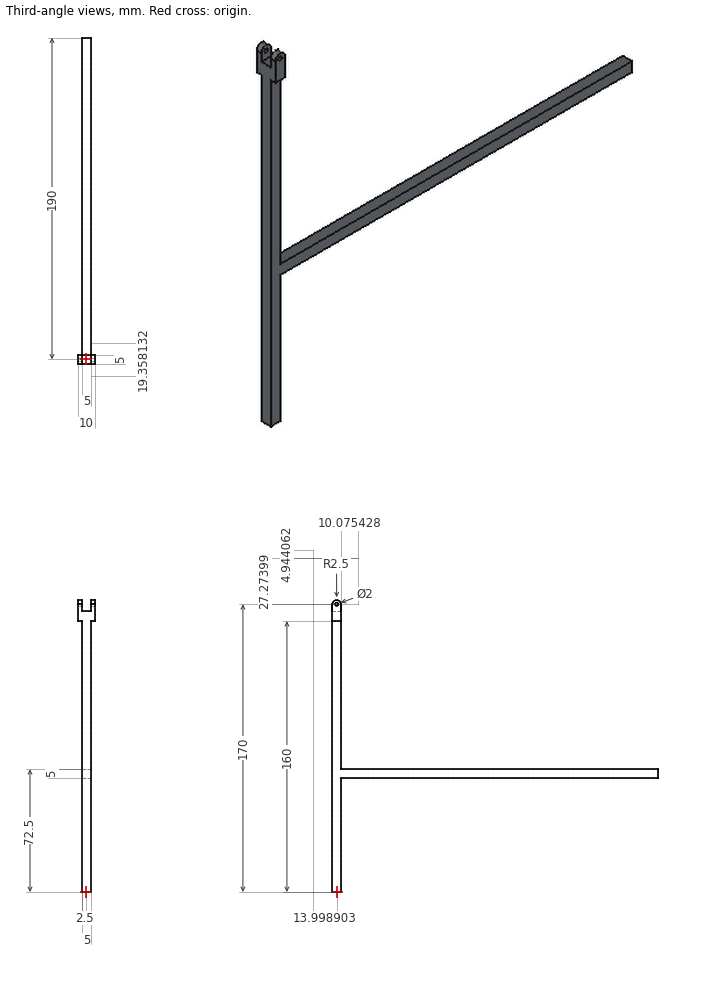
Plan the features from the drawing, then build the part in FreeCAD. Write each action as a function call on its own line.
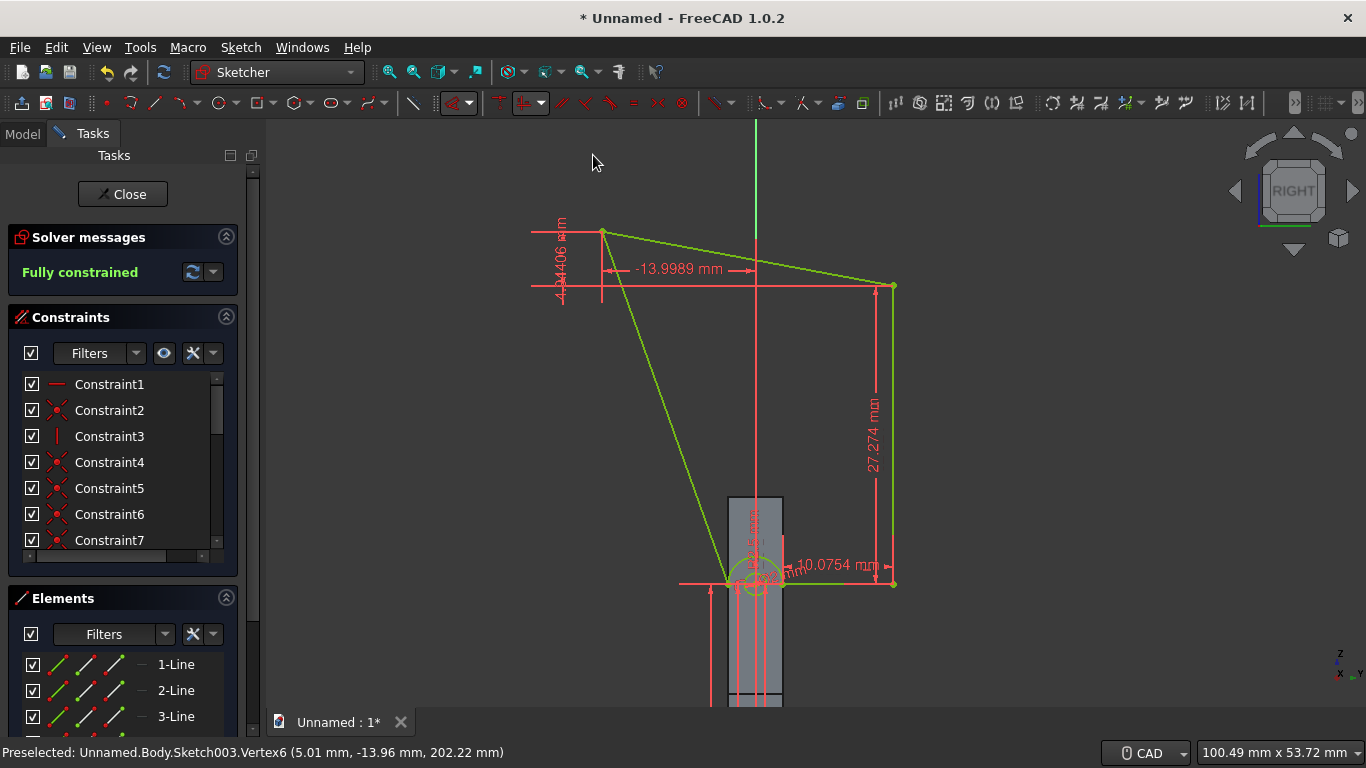
click(123, 194)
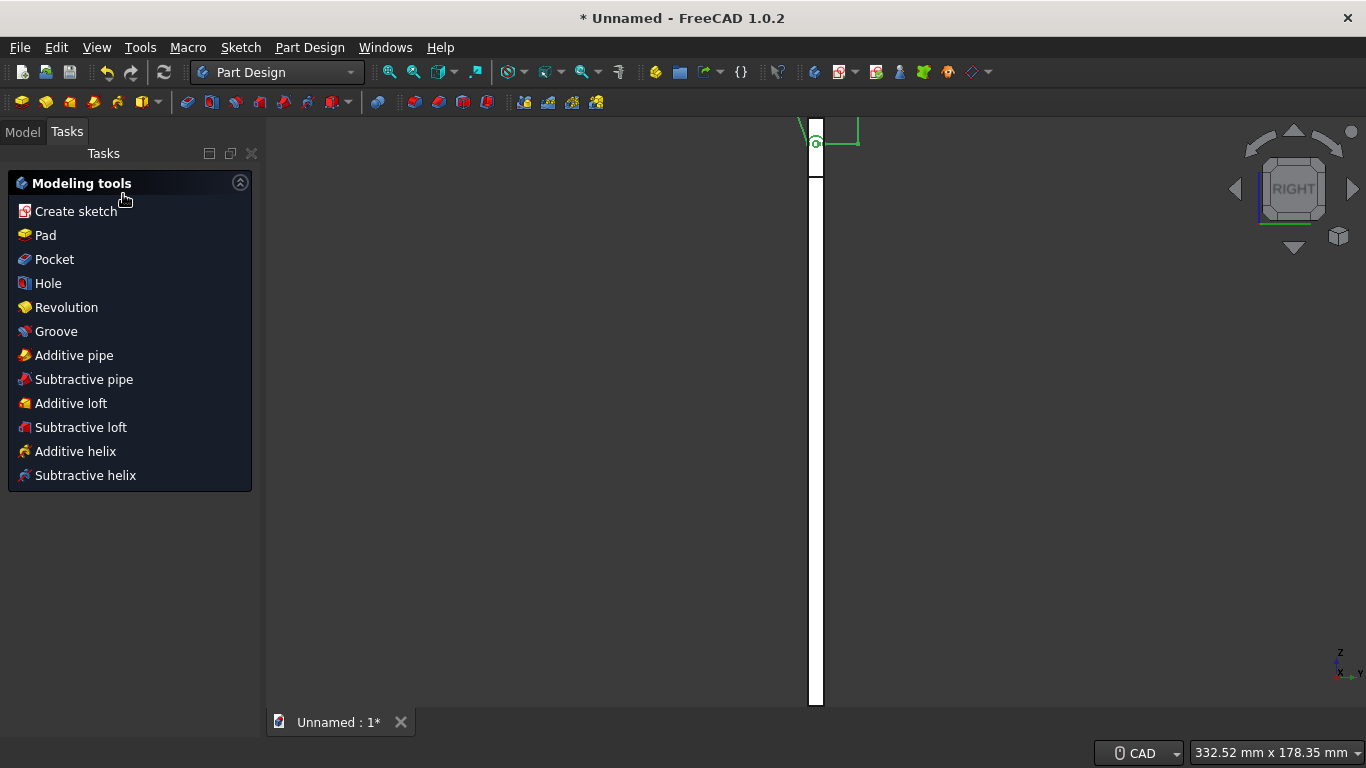
click(188, 102)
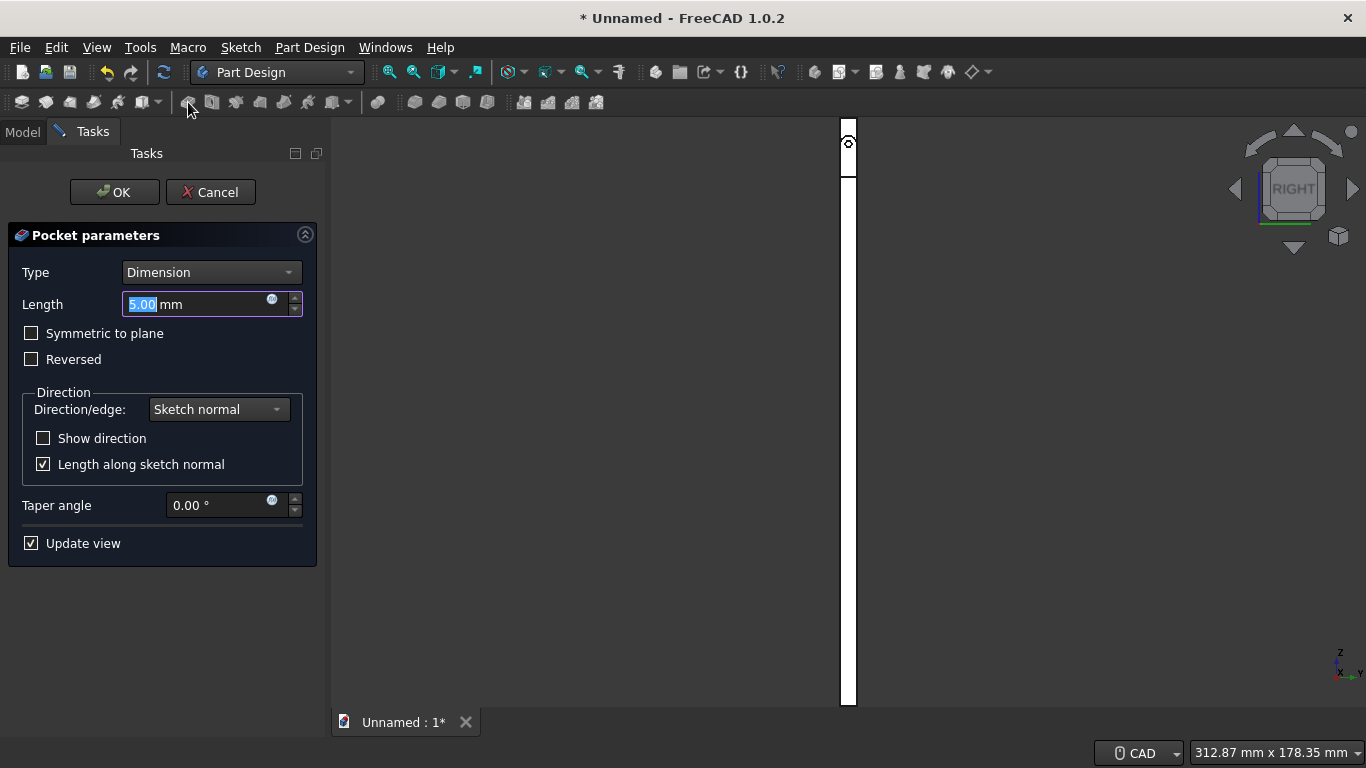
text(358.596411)
key(Tab)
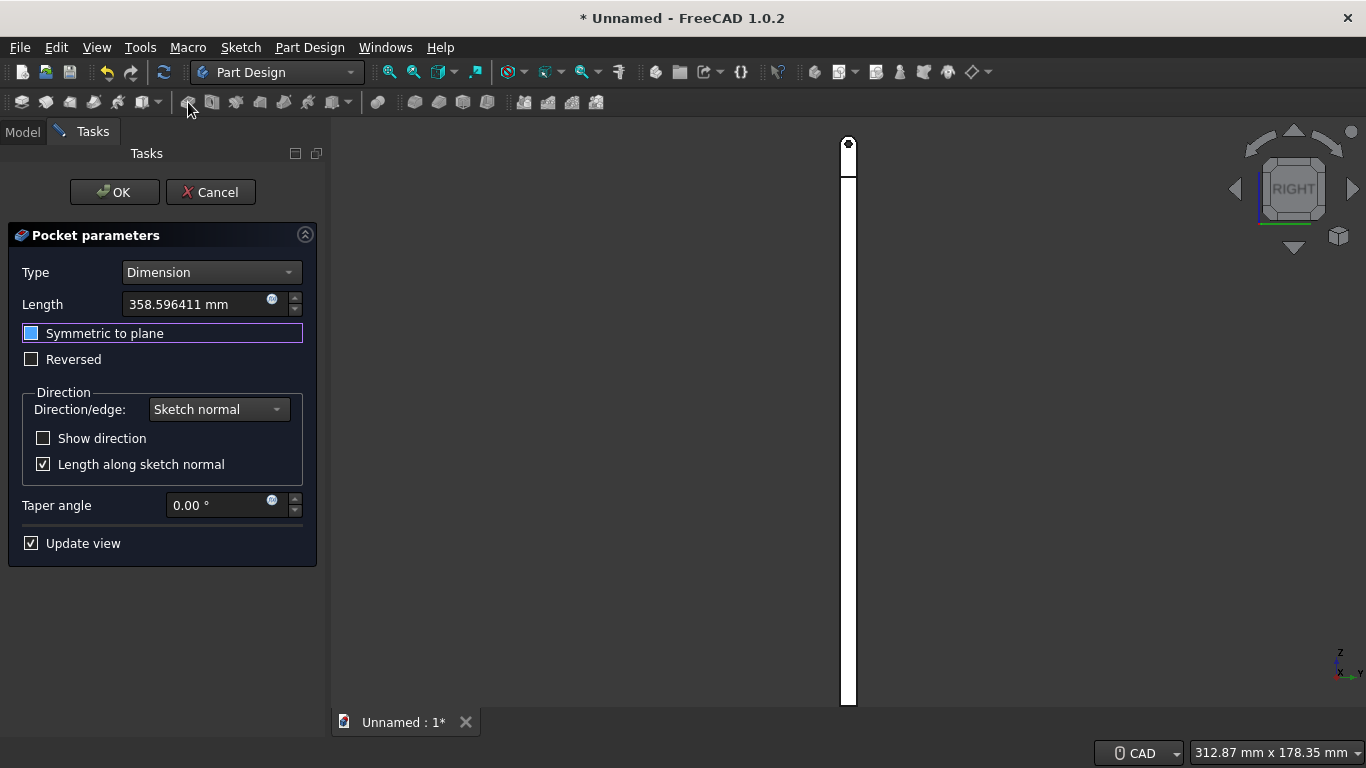
click(30, 333)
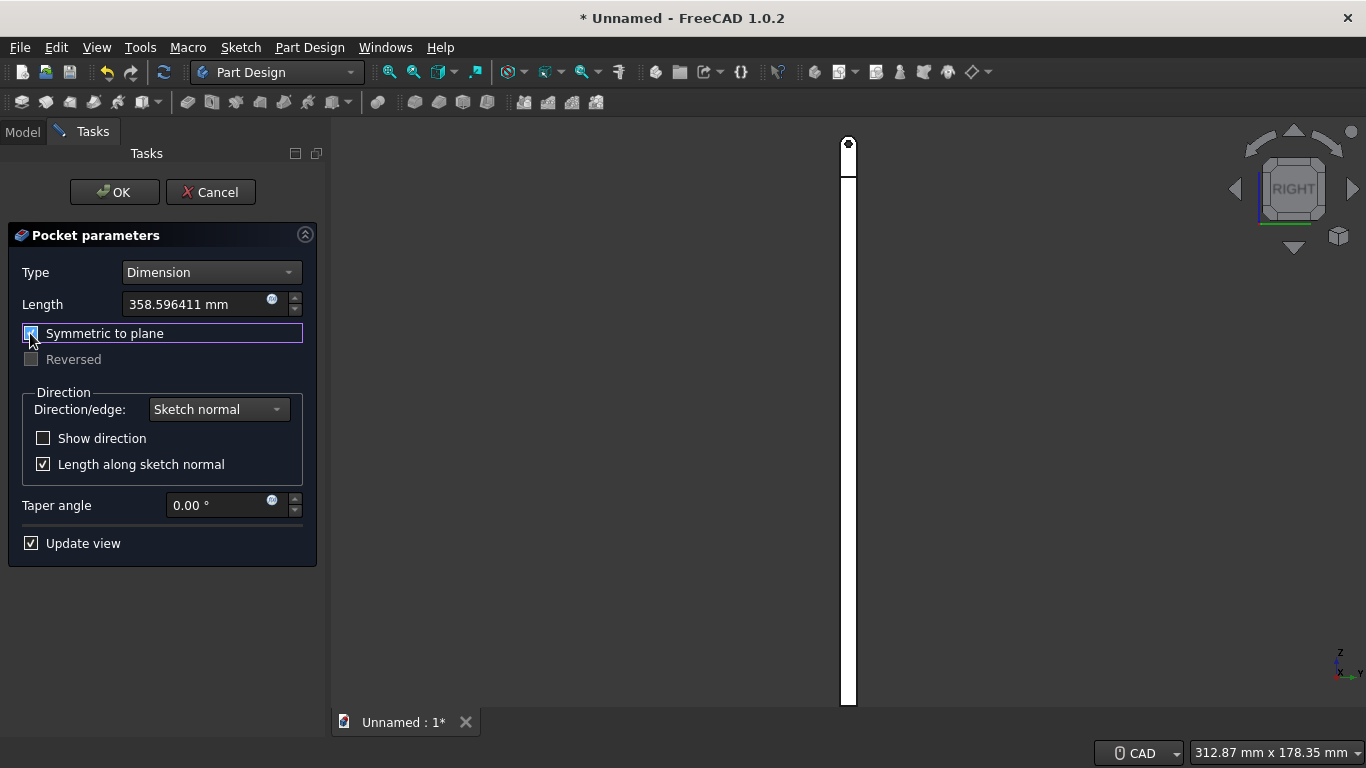
click(115, 192)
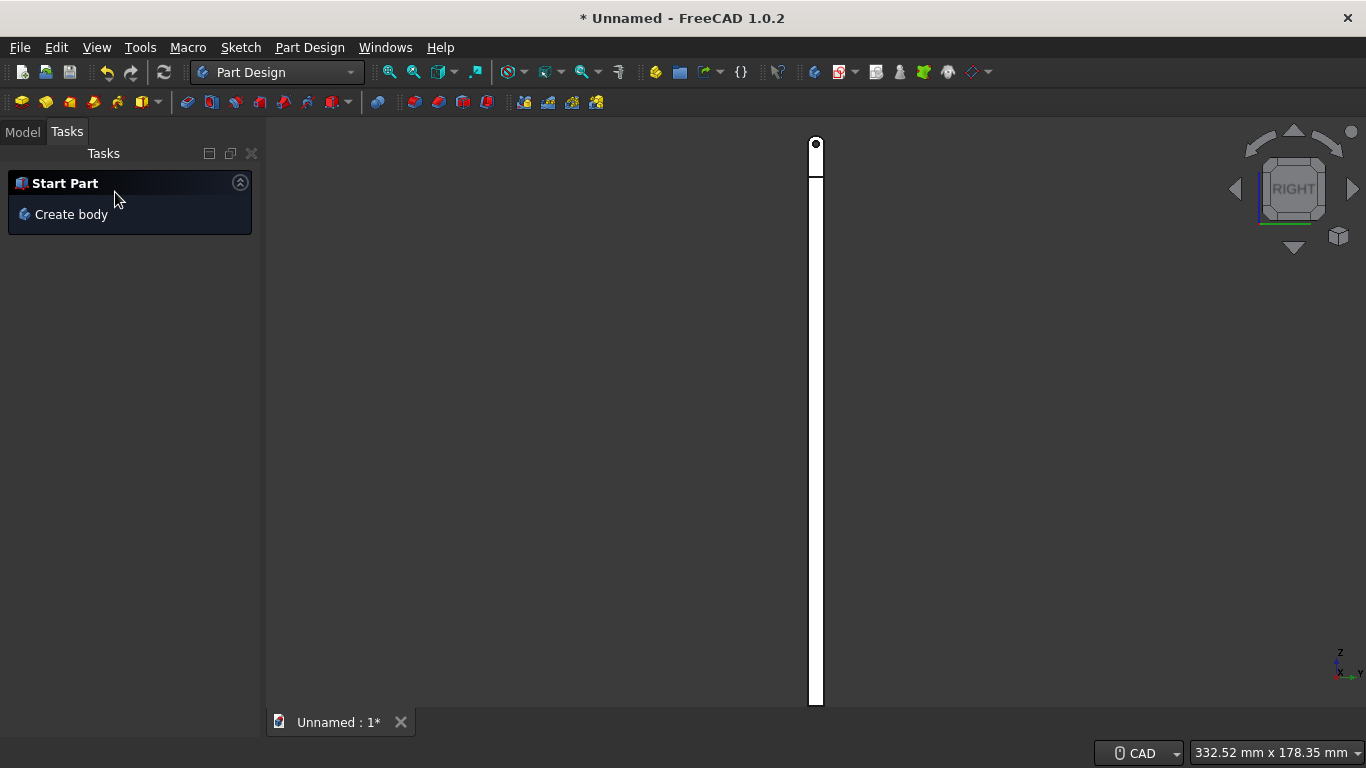
click(840, 72)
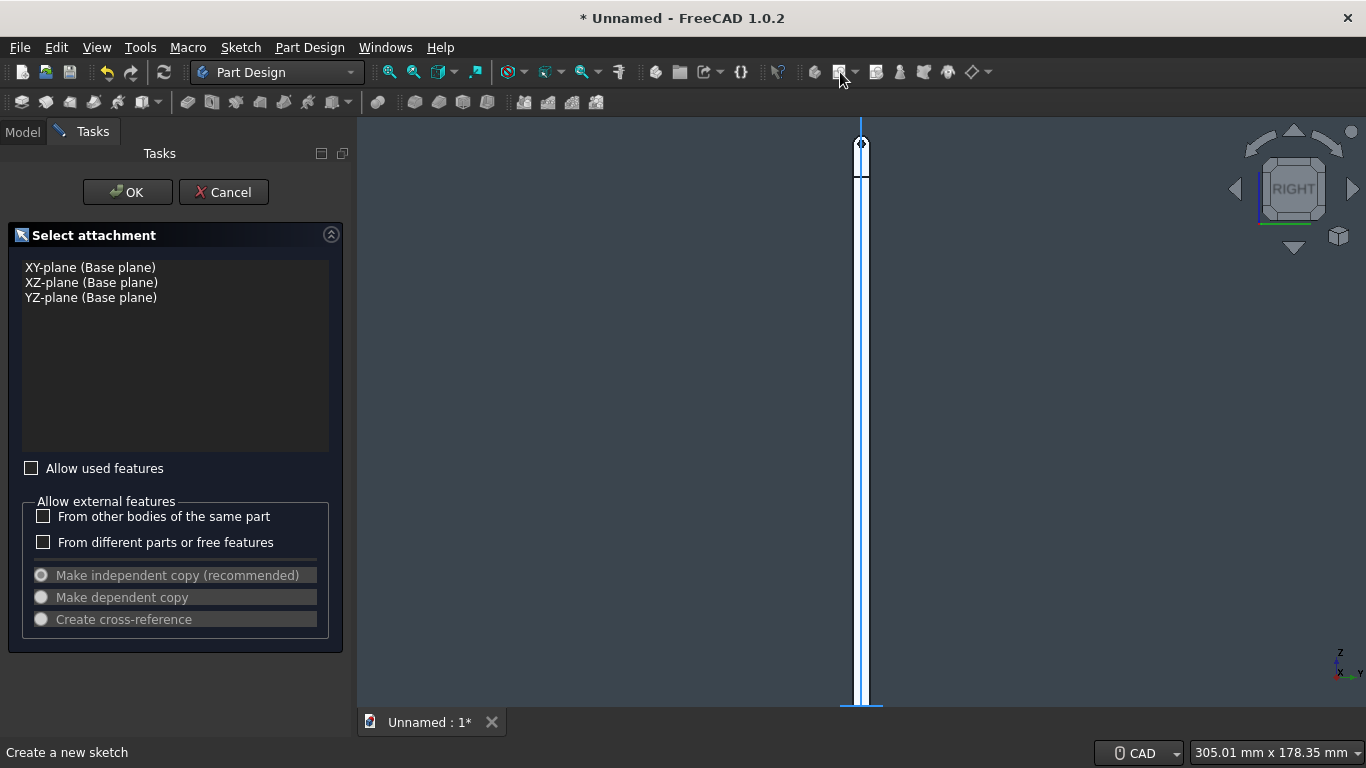
click(82, 282)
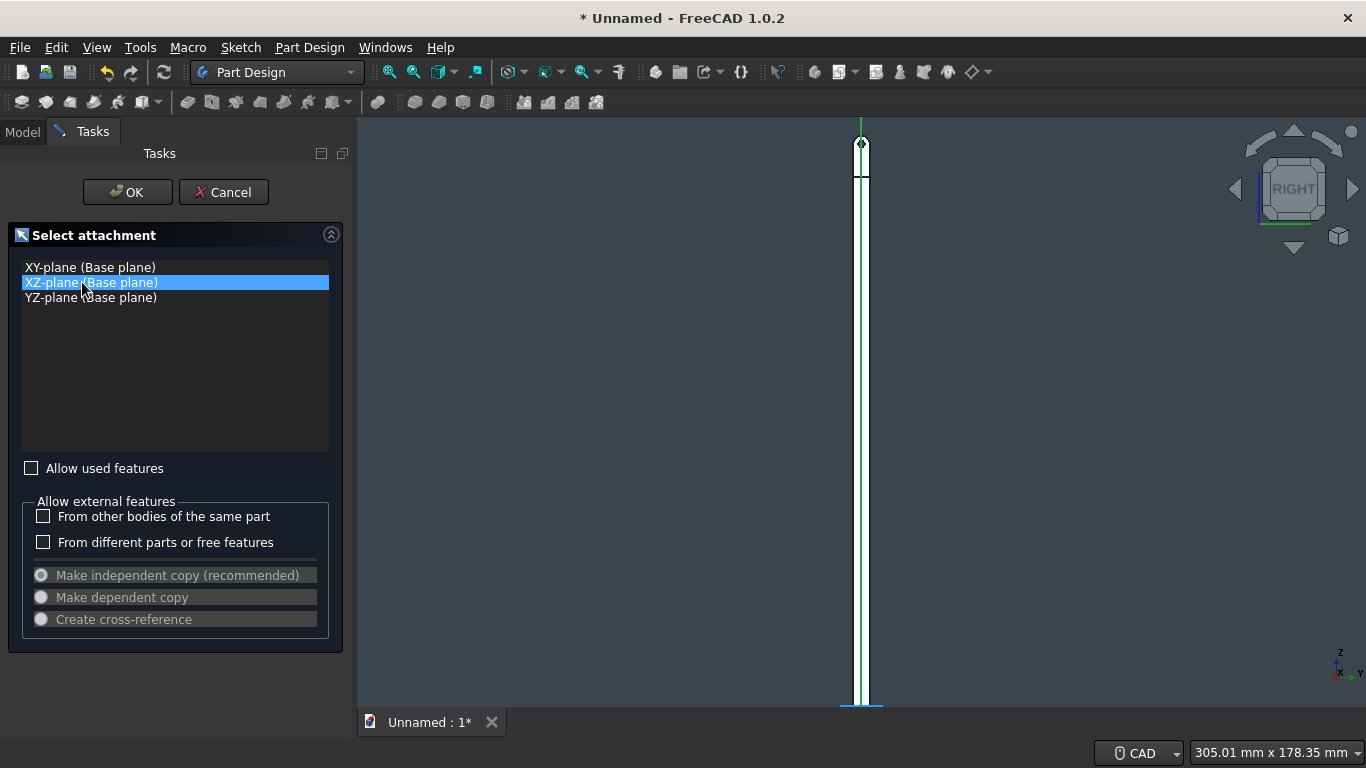
click(128, 192)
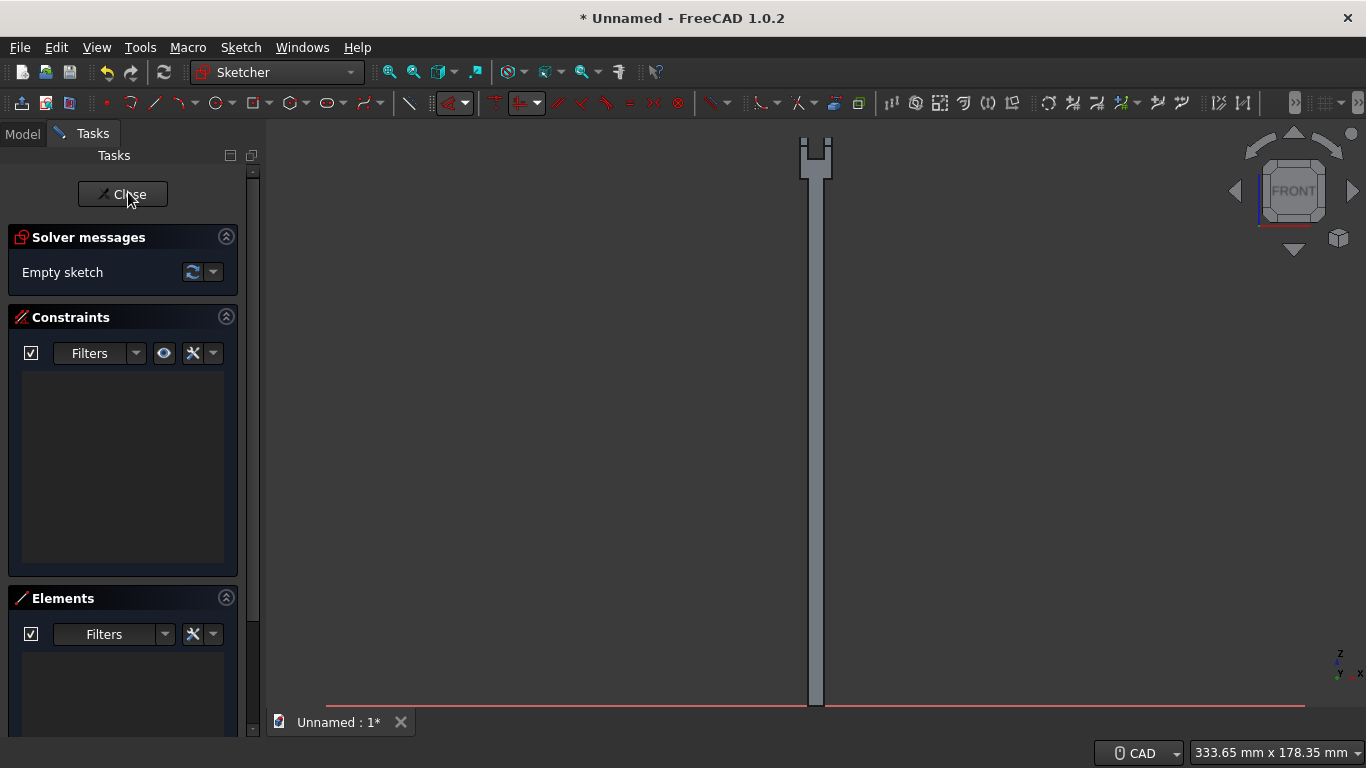
click(70, 104)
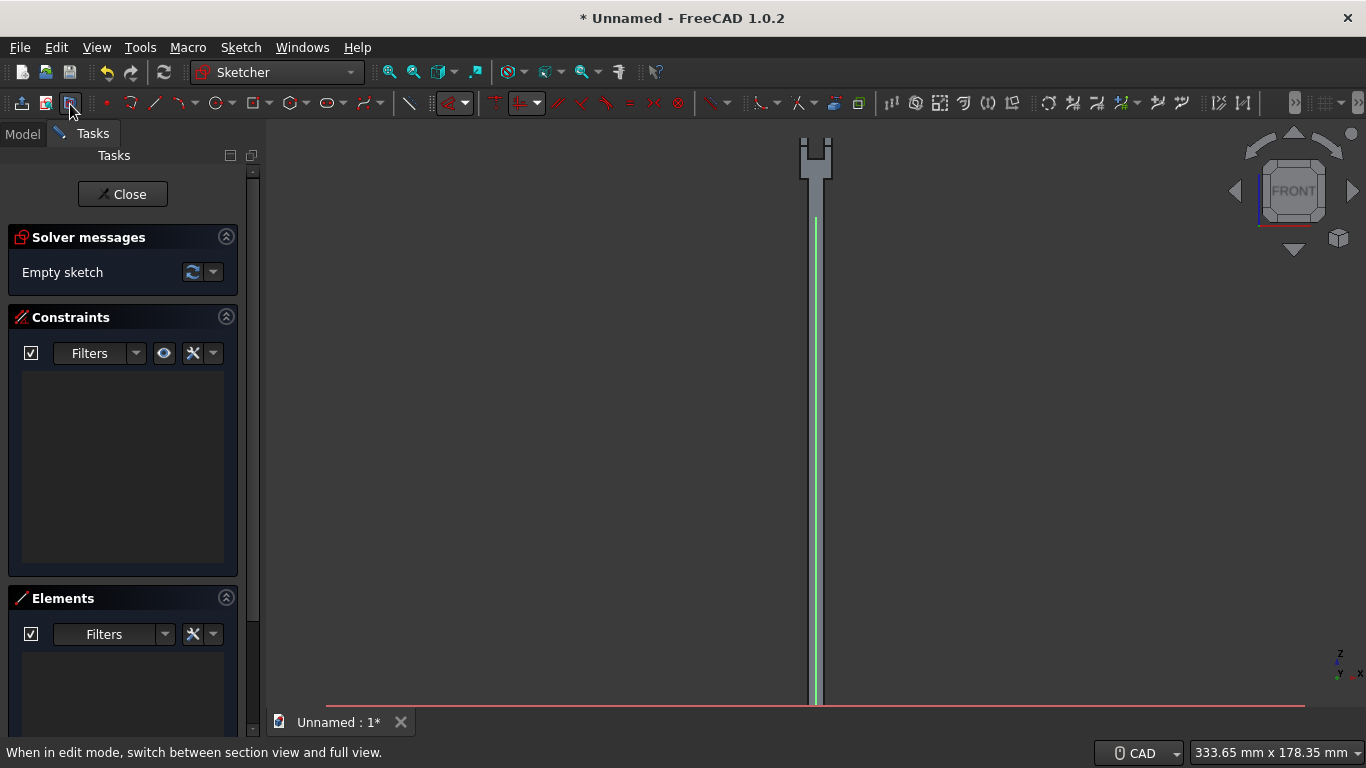
scroll(820, 479, up, 15)